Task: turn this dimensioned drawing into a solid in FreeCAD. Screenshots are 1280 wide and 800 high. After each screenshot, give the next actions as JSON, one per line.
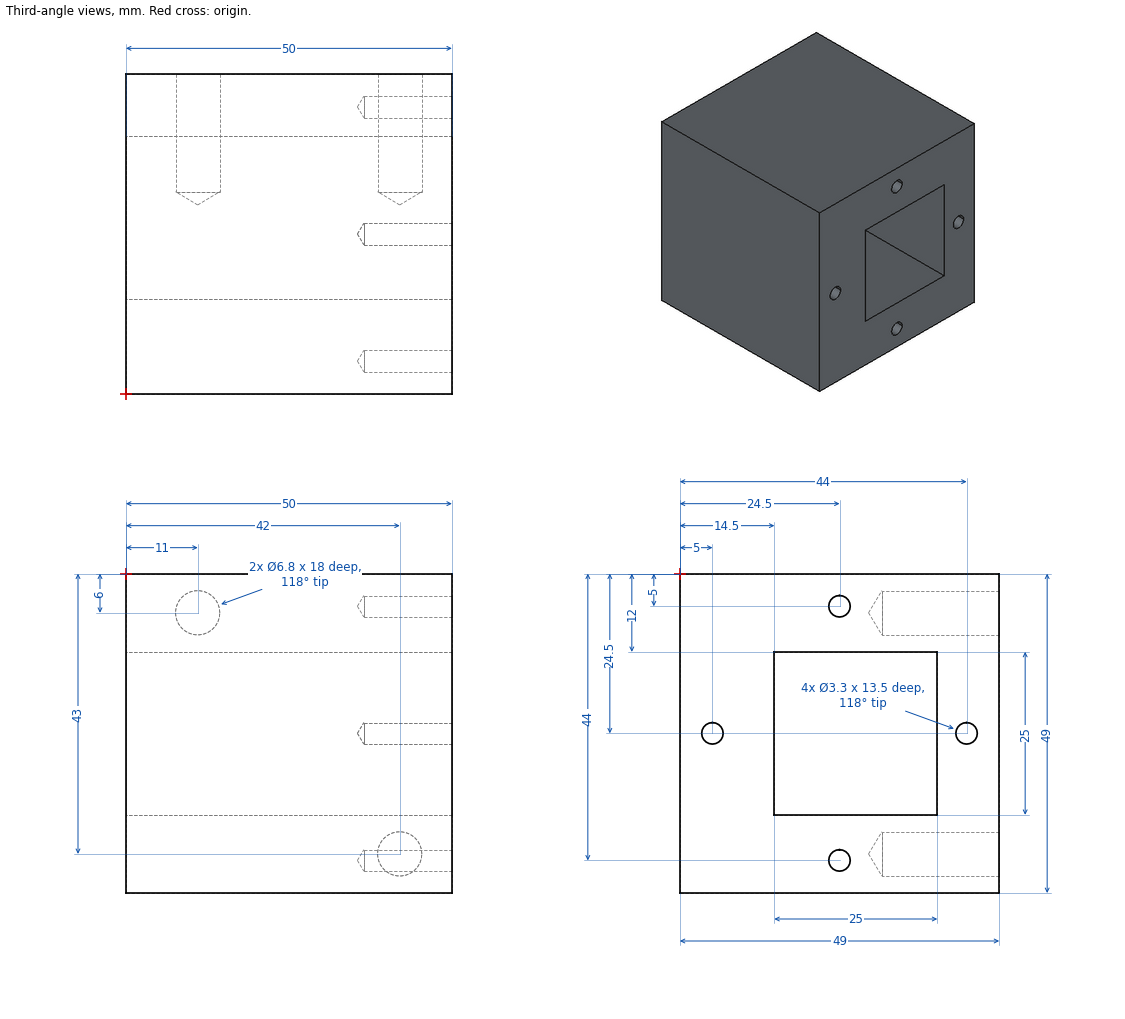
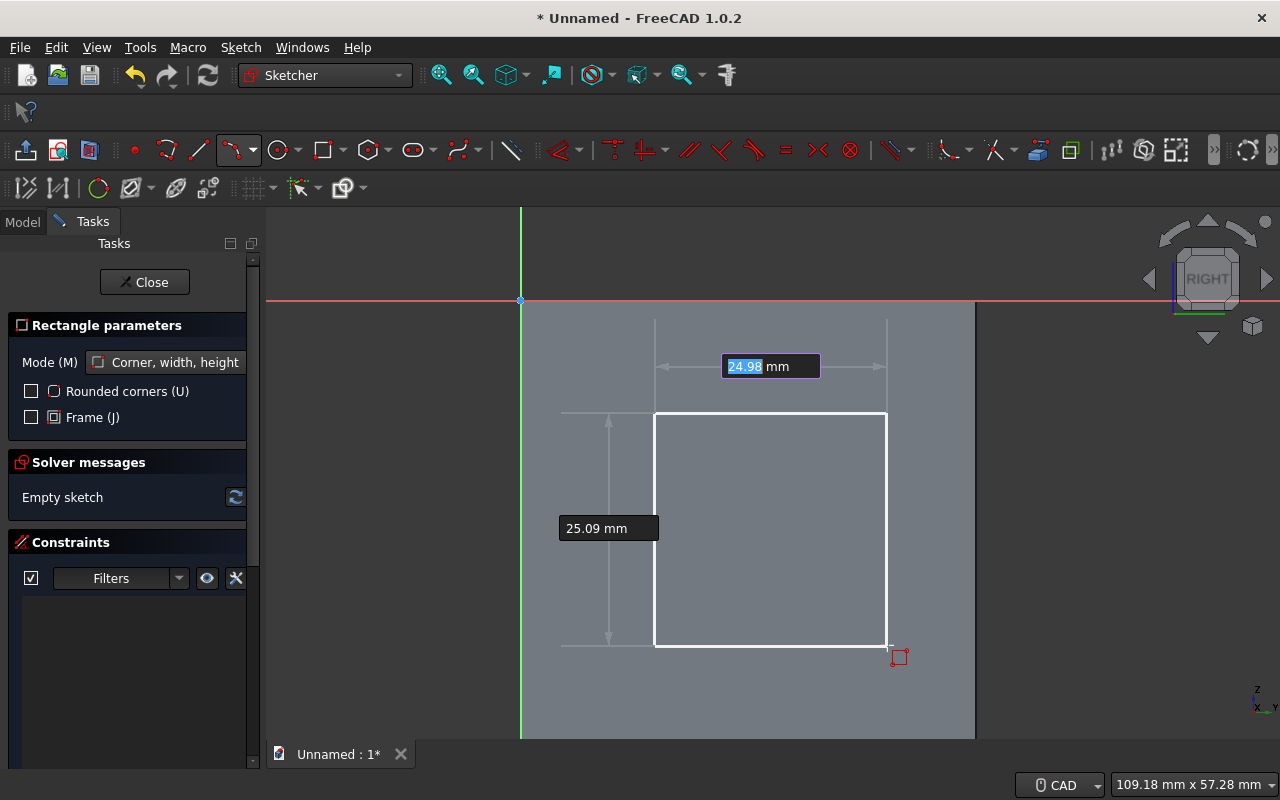
{"action": "type", "text": "25"}
{"action": "key", "text": "Tab"}
{"action": "type", "text": "25"}
{"action": "key", "text": "Return"}
{"action": "key", "text": "Escape"}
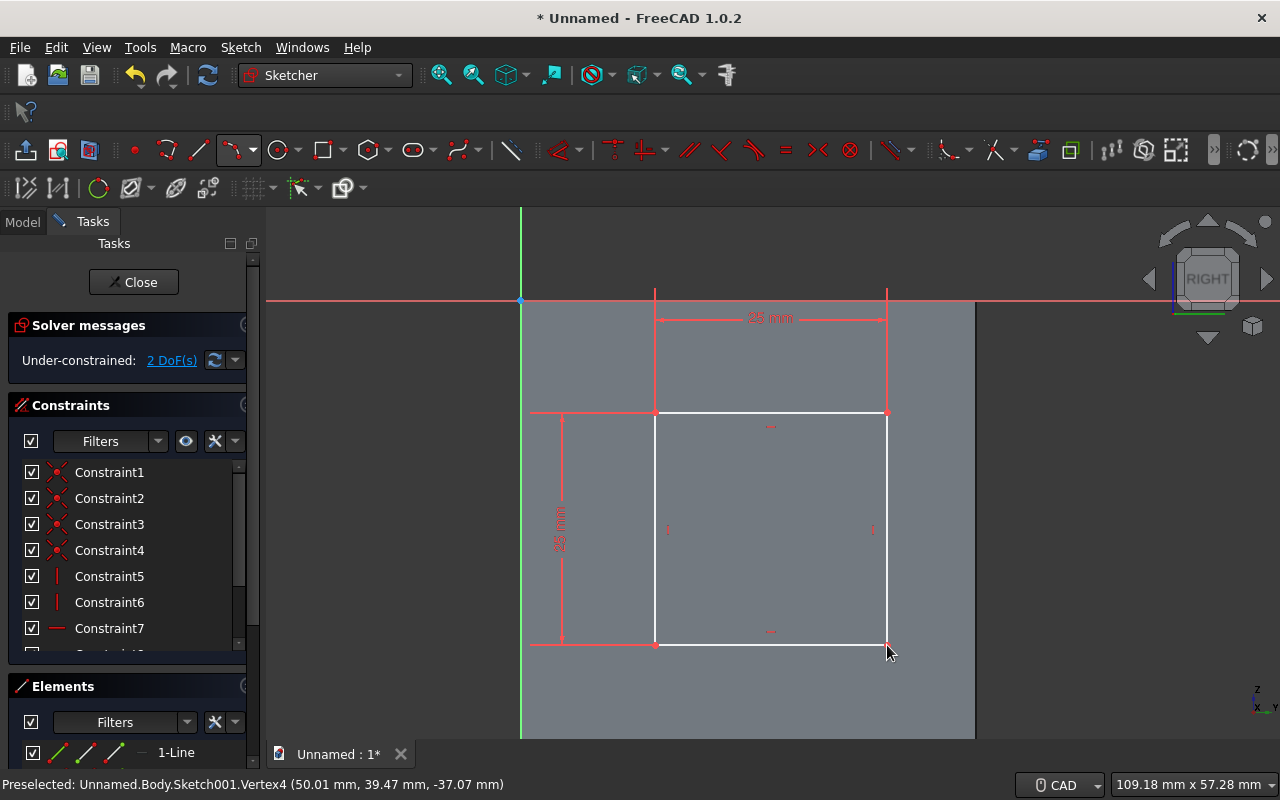
{"action": "key", "text": "d"}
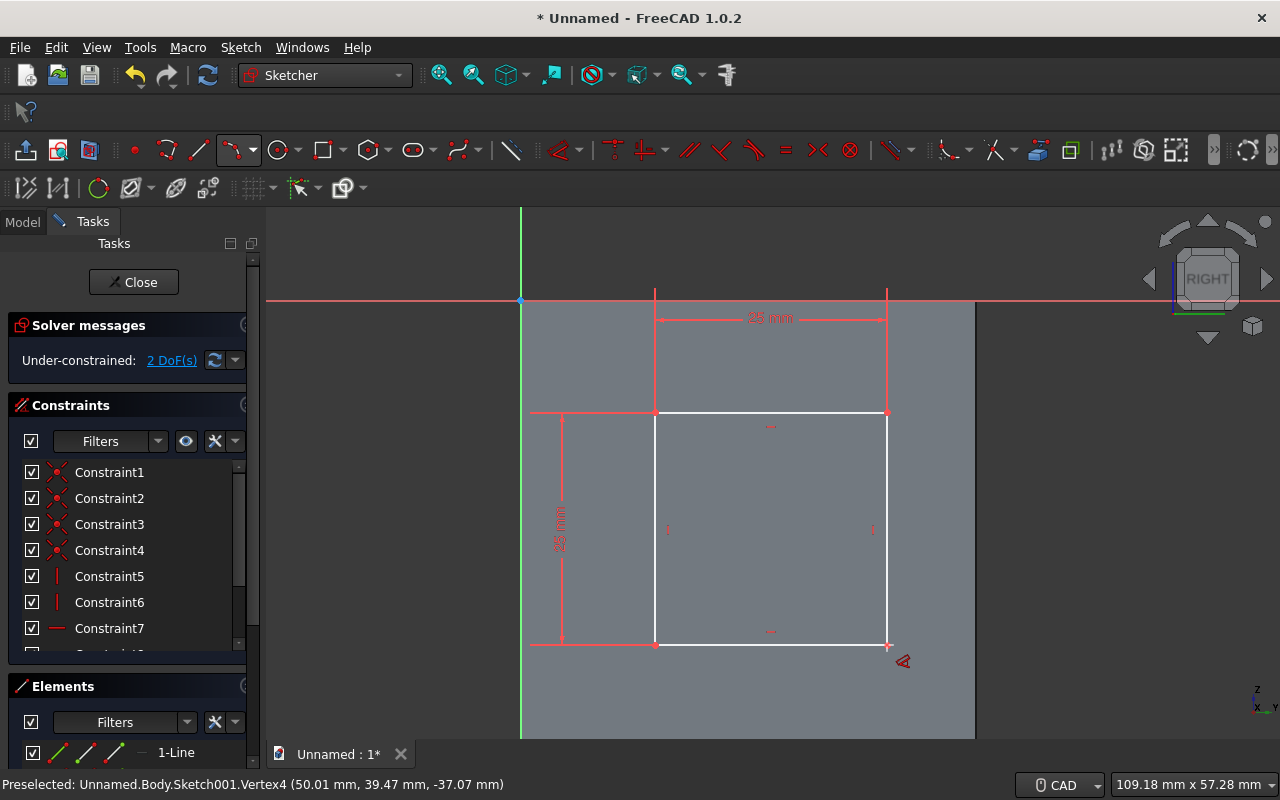
{"action": "left_click", "coordinate": [655, 413]}
{"action": "left_click", "coordinate": [487, 357]}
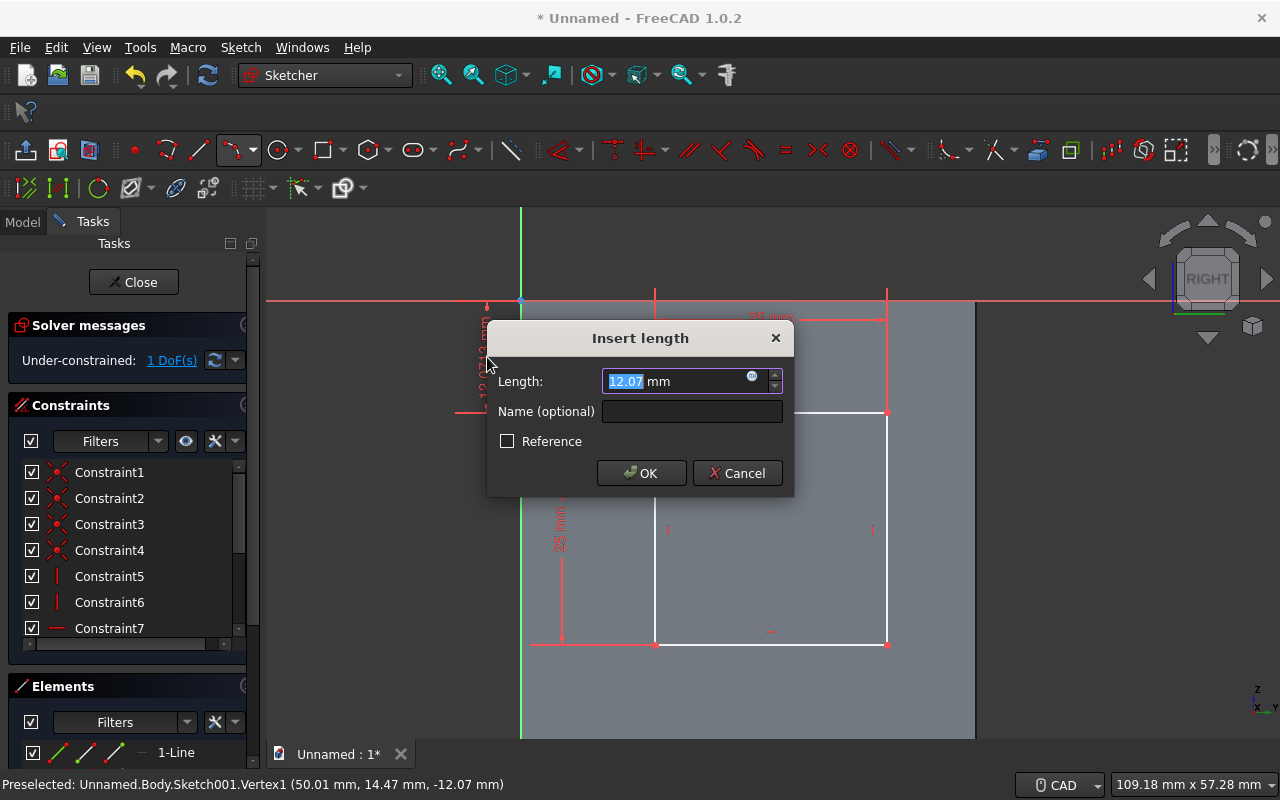
{"action": "type", "text": "12"}
{"action": "key", "text": "Return"}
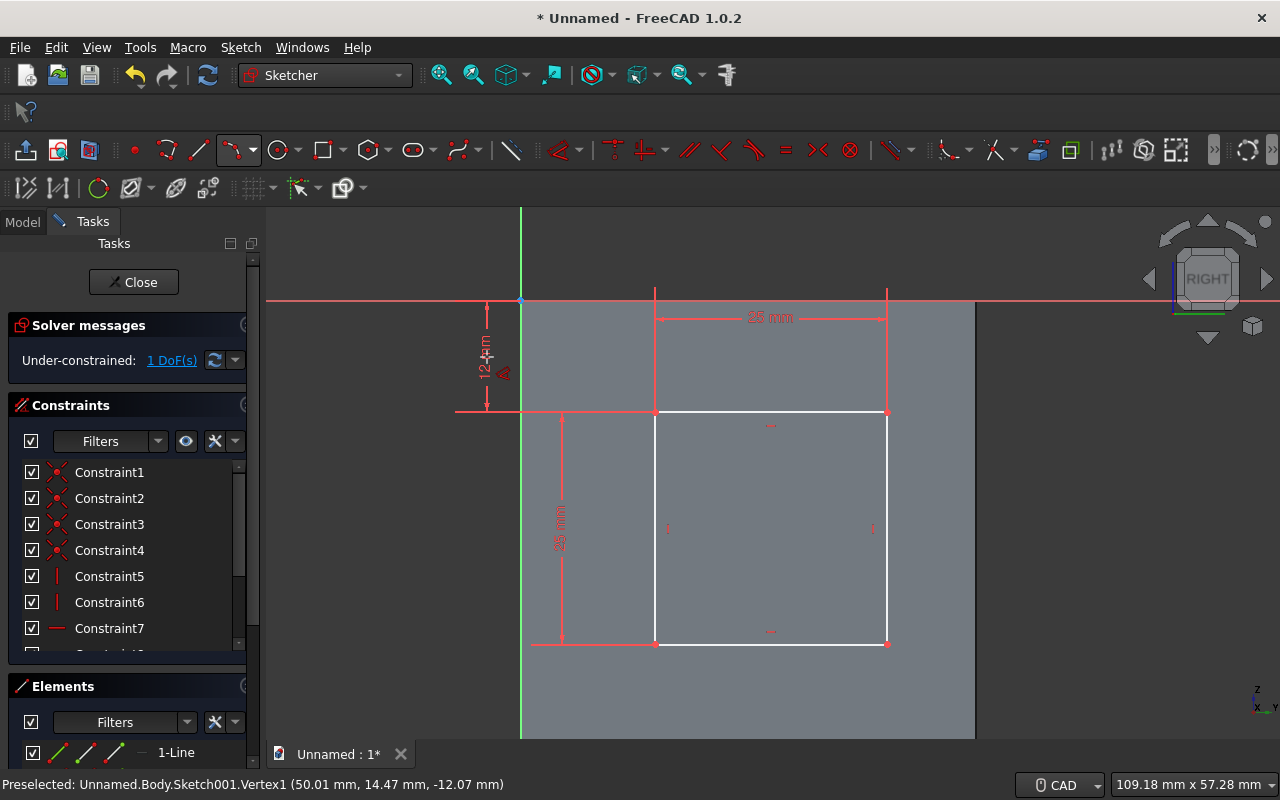
{"action": "left_click", "coordinate": [655, 412]}
{"action": "left_click", "coordinate": [588, 267]}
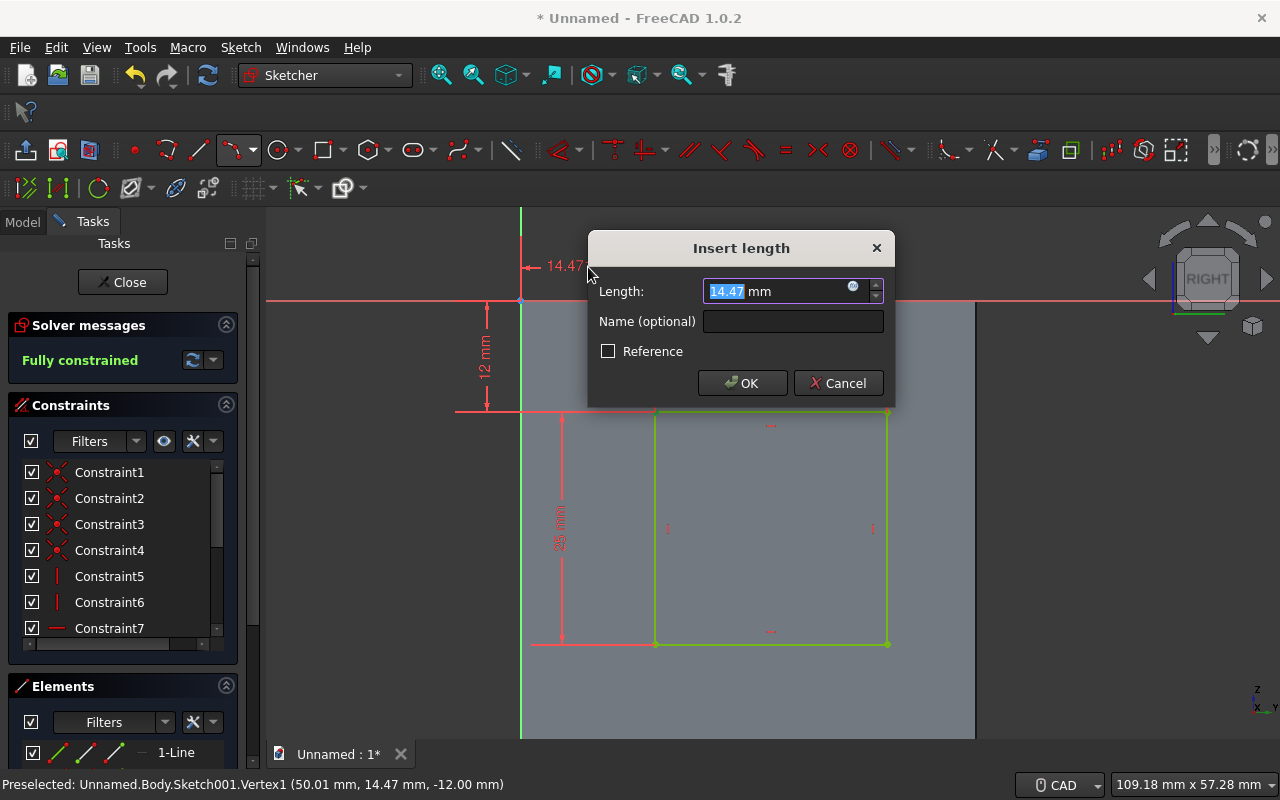
{"action": "type", "text": "14.5"}
{"action": "key", "text": "Return"}
{"action": "key", "text": "Escape"}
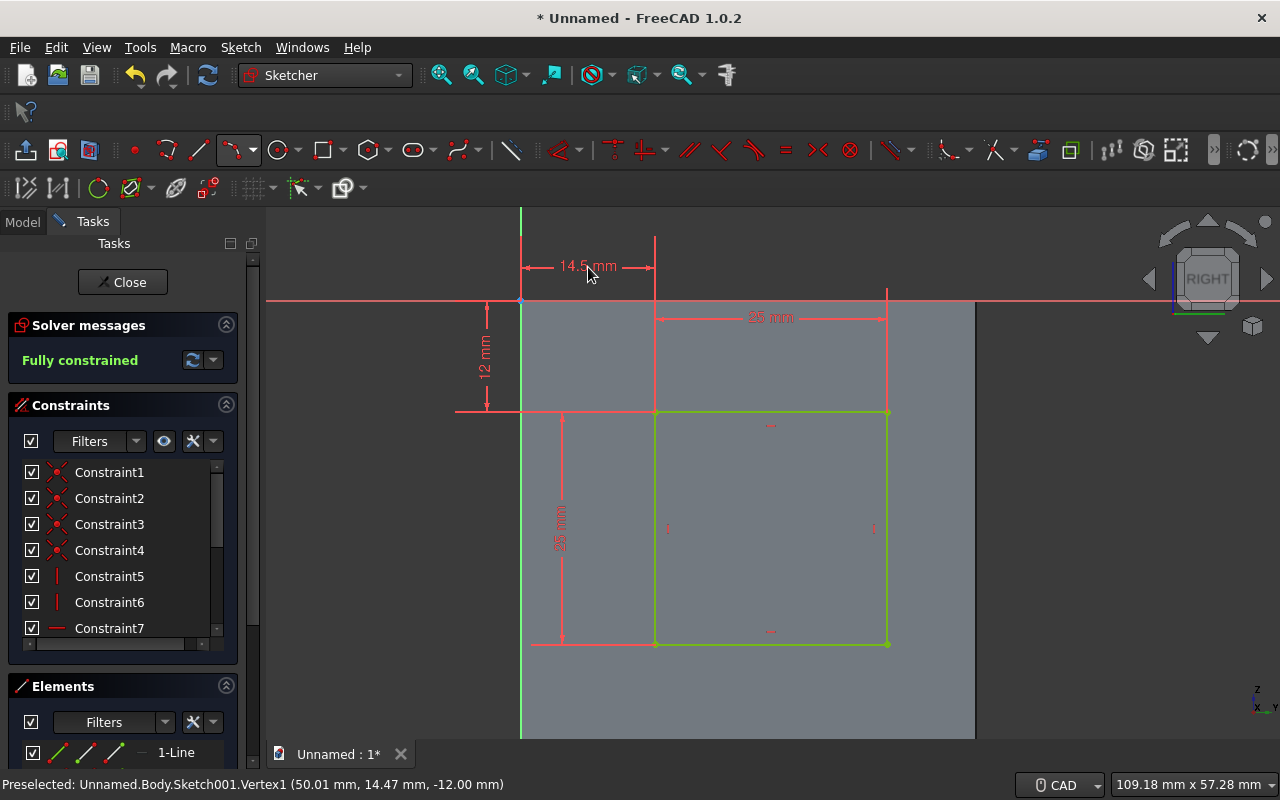
{"action": "left_click", "coordinate": [123, 282]}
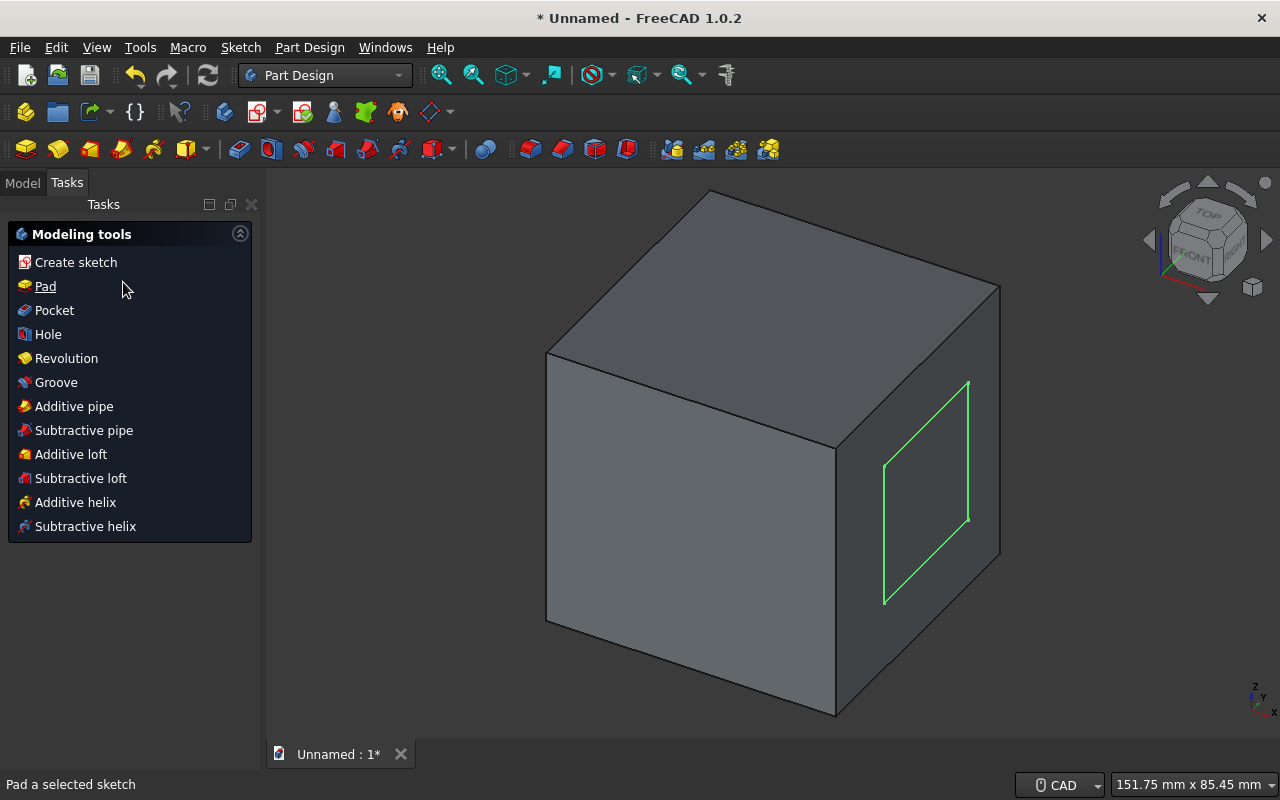
{"action": "left_click", "coordinate": [240, 150]}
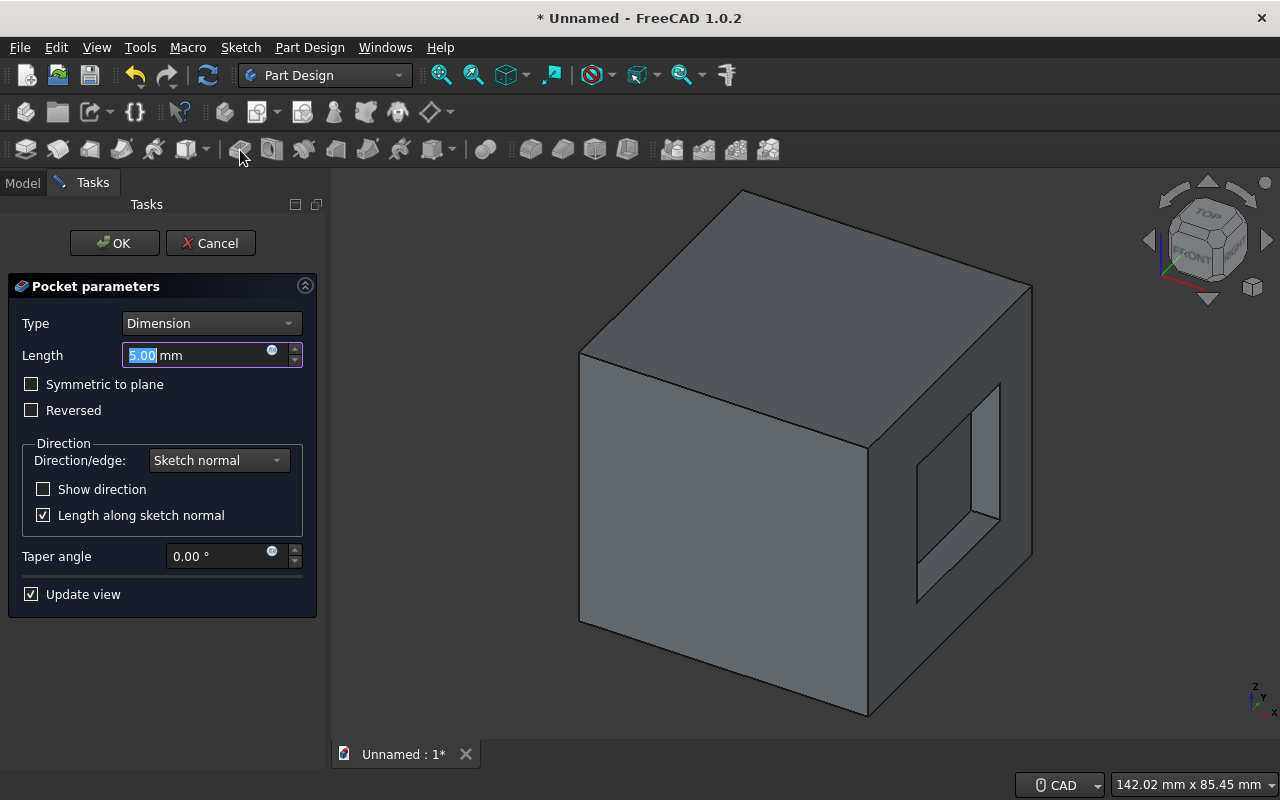
{"action": "type", "text": "50"}
{"action": "key", "text": "Tab"}